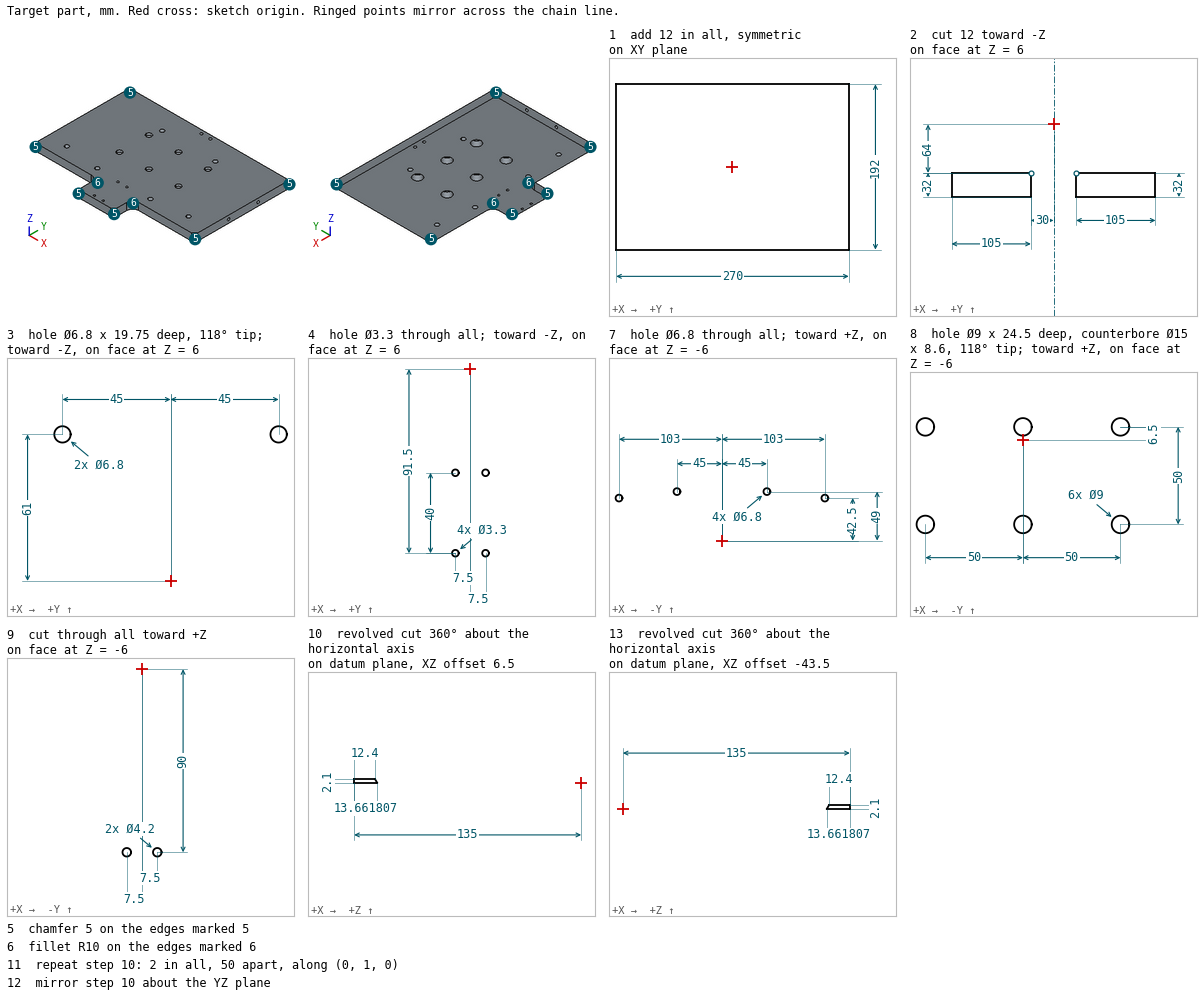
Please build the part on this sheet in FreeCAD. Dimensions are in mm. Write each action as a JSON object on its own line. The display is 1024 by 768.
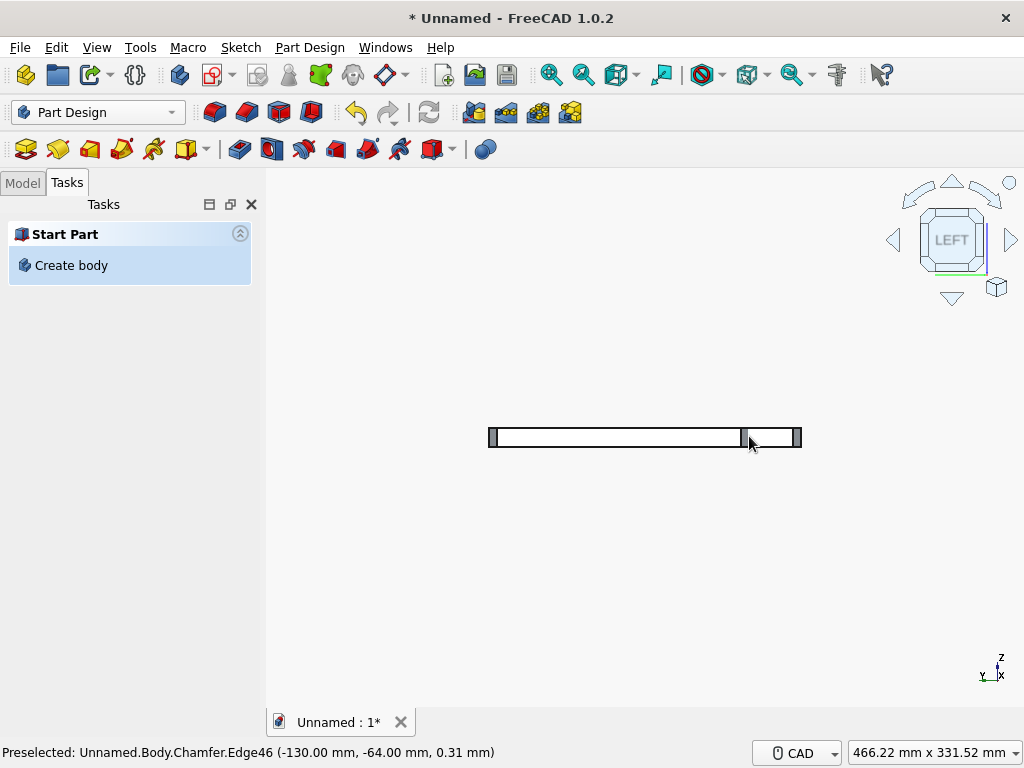
{"action": "key", "text": "v 3"}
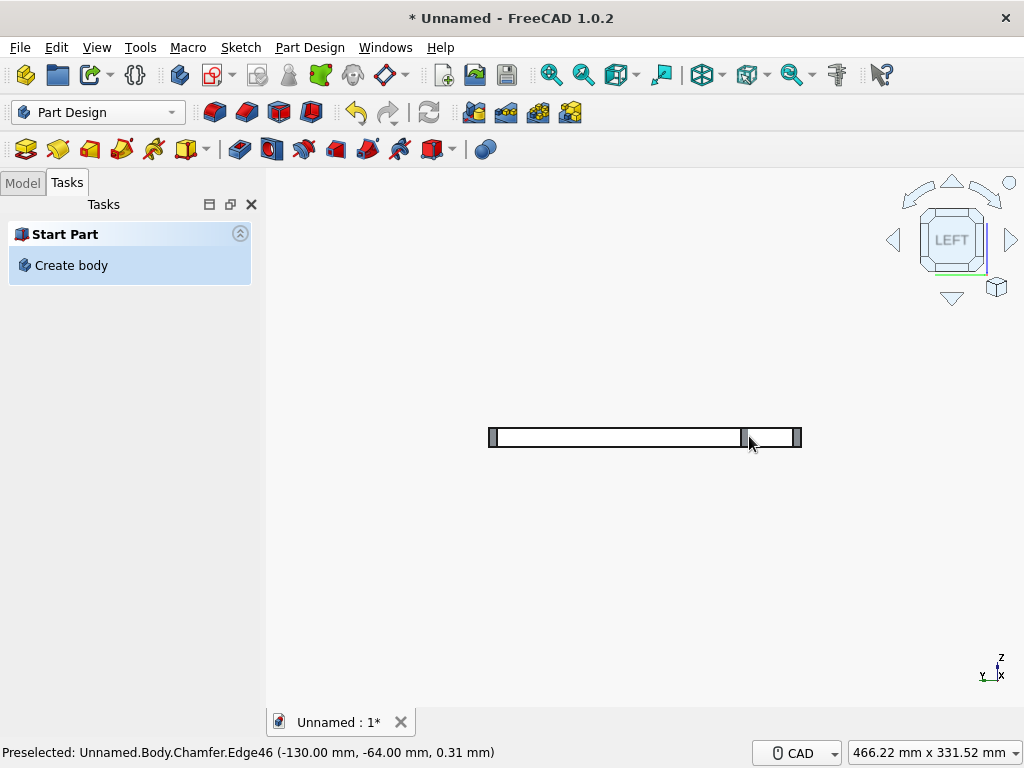
{"action": "key", "text": "0"}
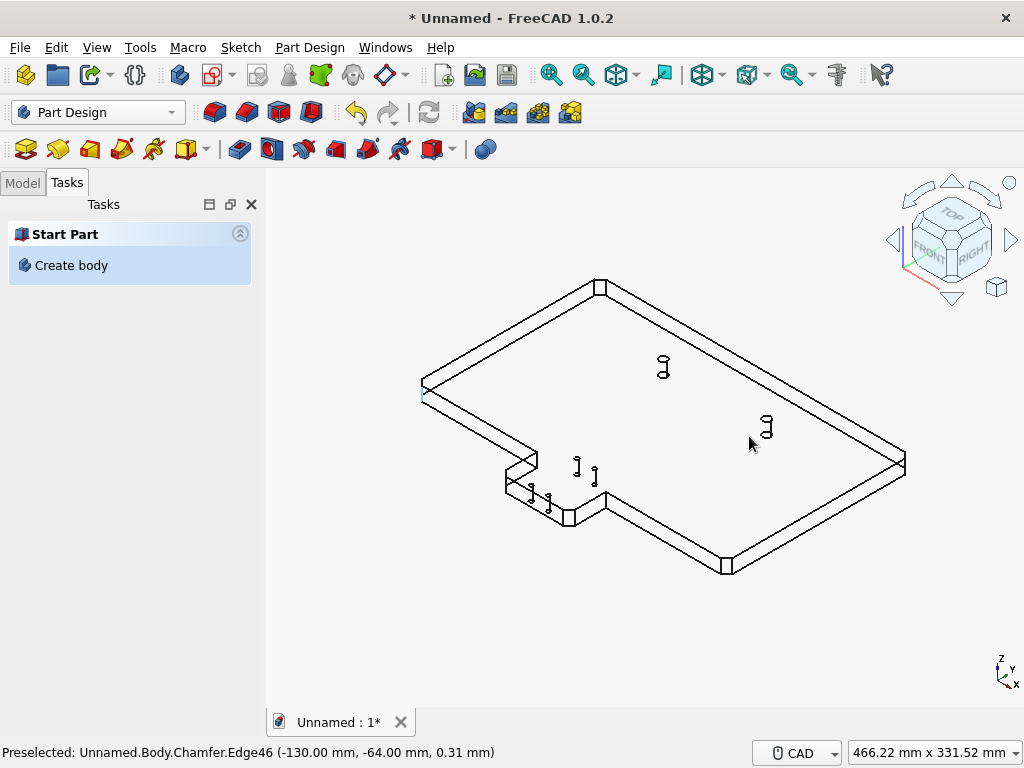
{"action": "left_click", "coordinate": [537, 459]}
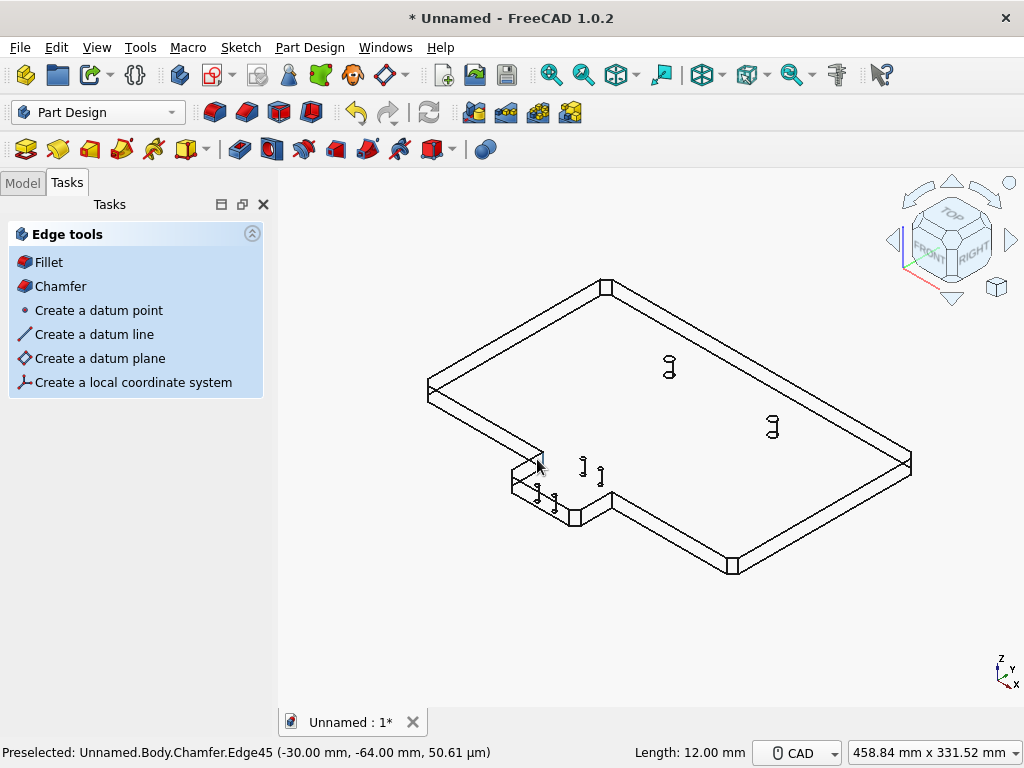
{"action": "left_click", "coordinate": [612, 499], "text": "ctrl"}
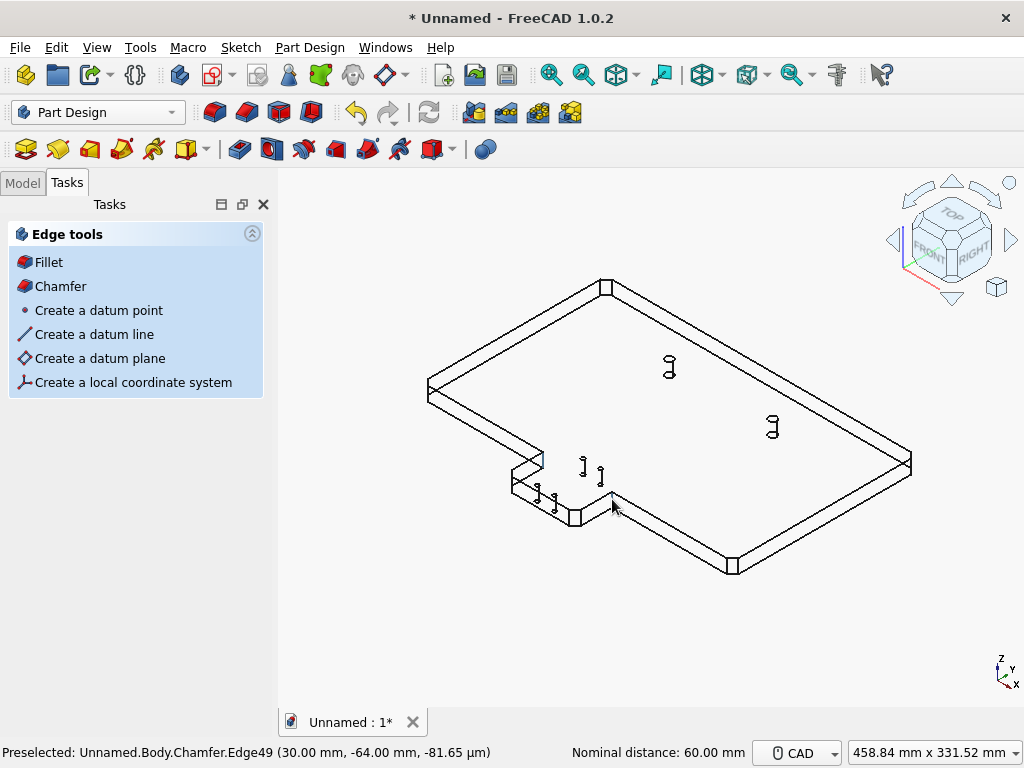
{"action": "key", "text": "v 1"}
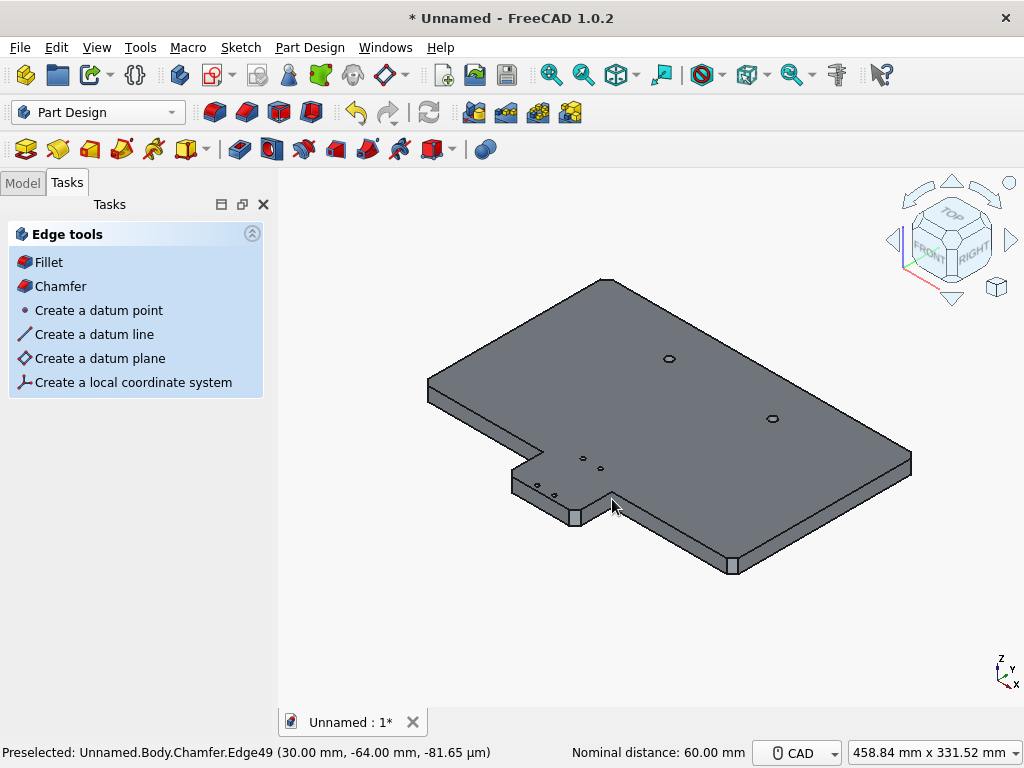
{"action": "left_click", "coordinate": [216, 112]}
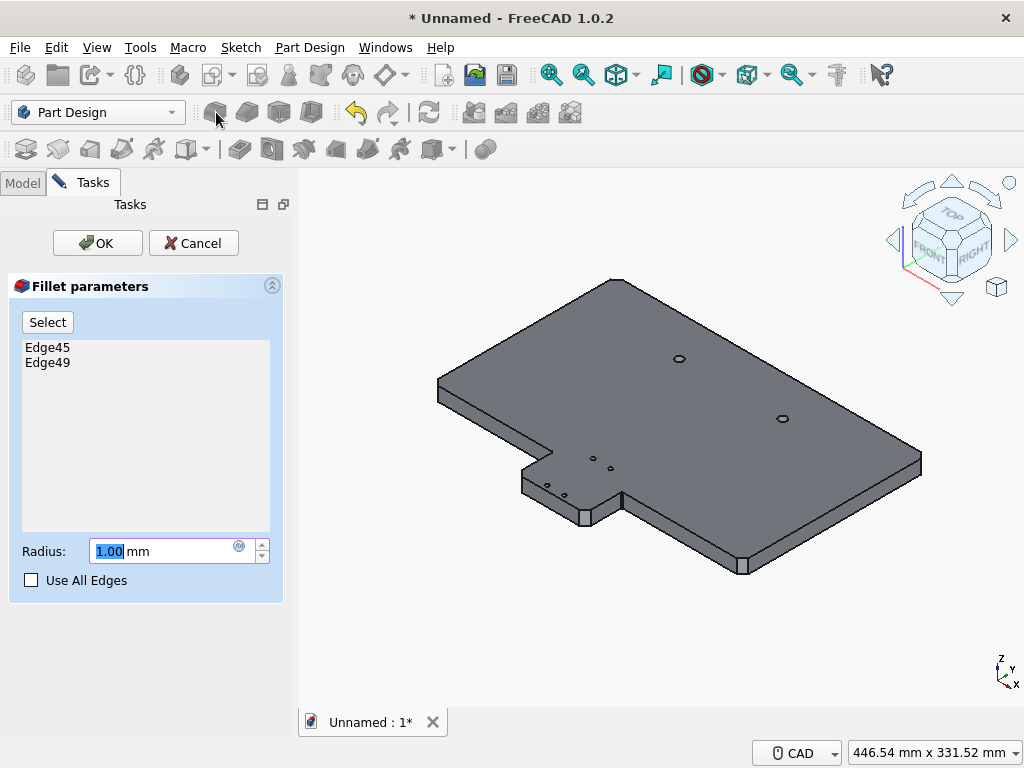
{"action": "type", "text": "10"}
{"action": "key", "text": "Tab"}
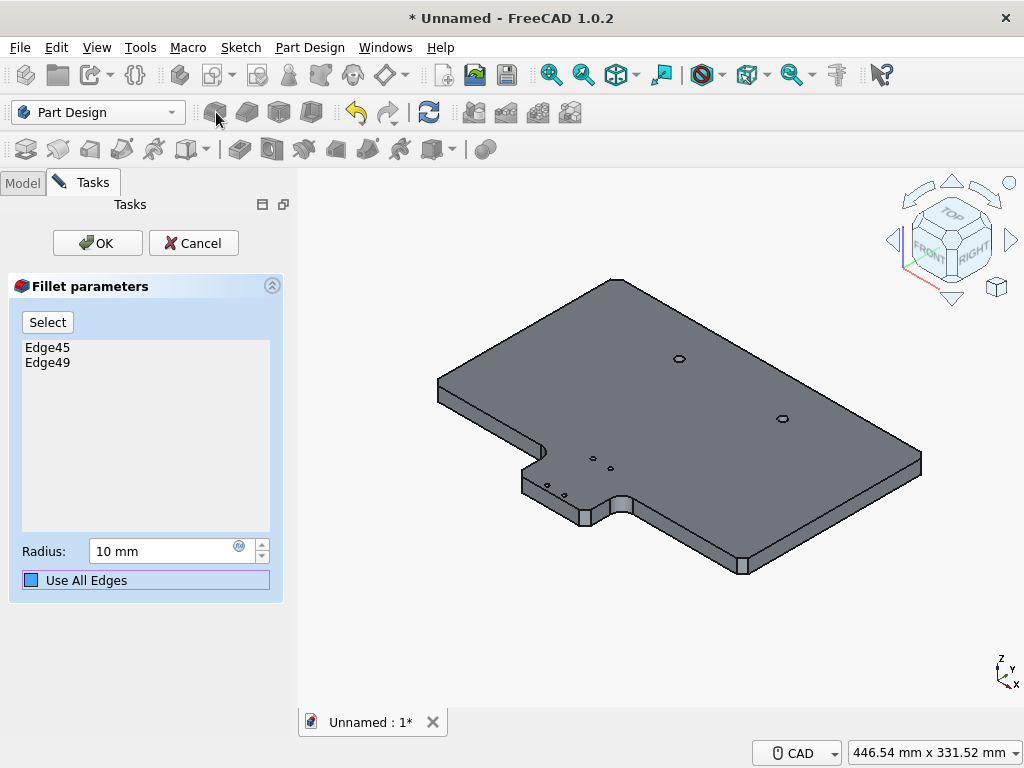
{"action": "left_click", "coordinate": [98, 243]}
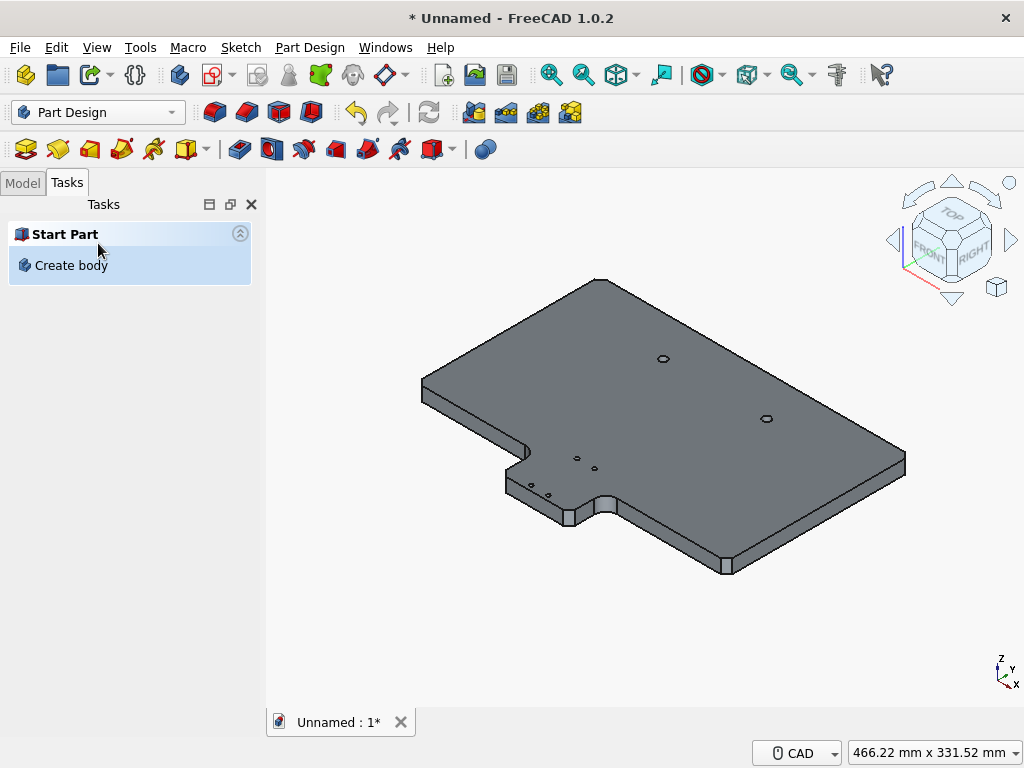
{"action": "key", "text": "5"}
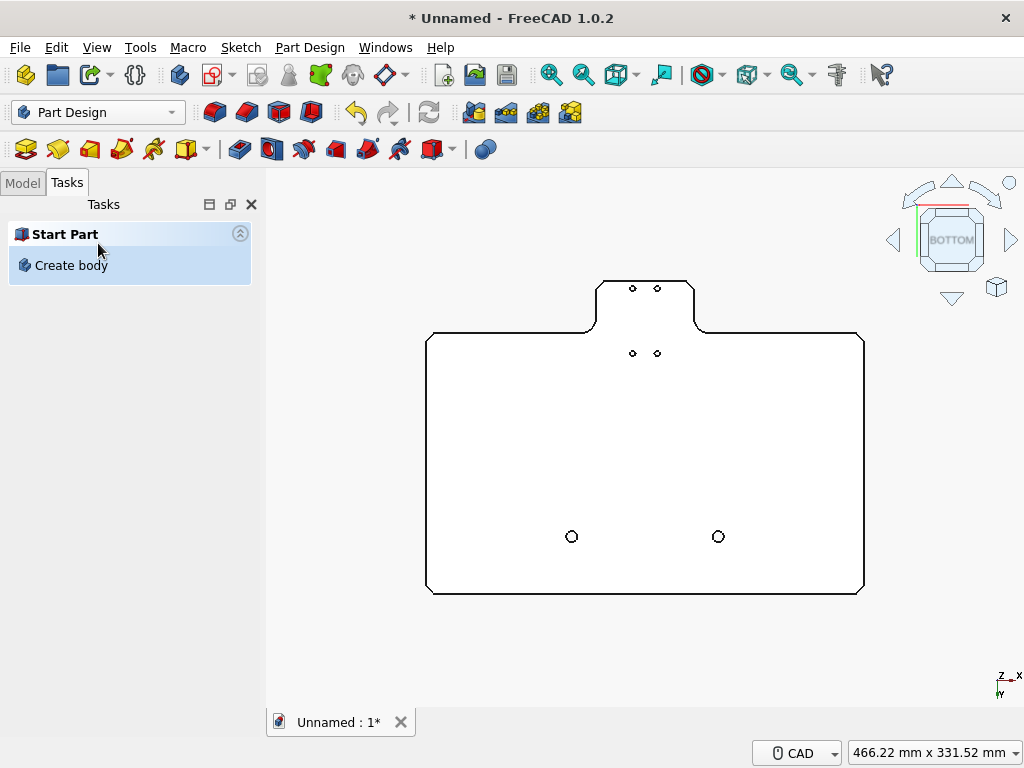
{"action": "left_click", "coordinate": [582, 436]}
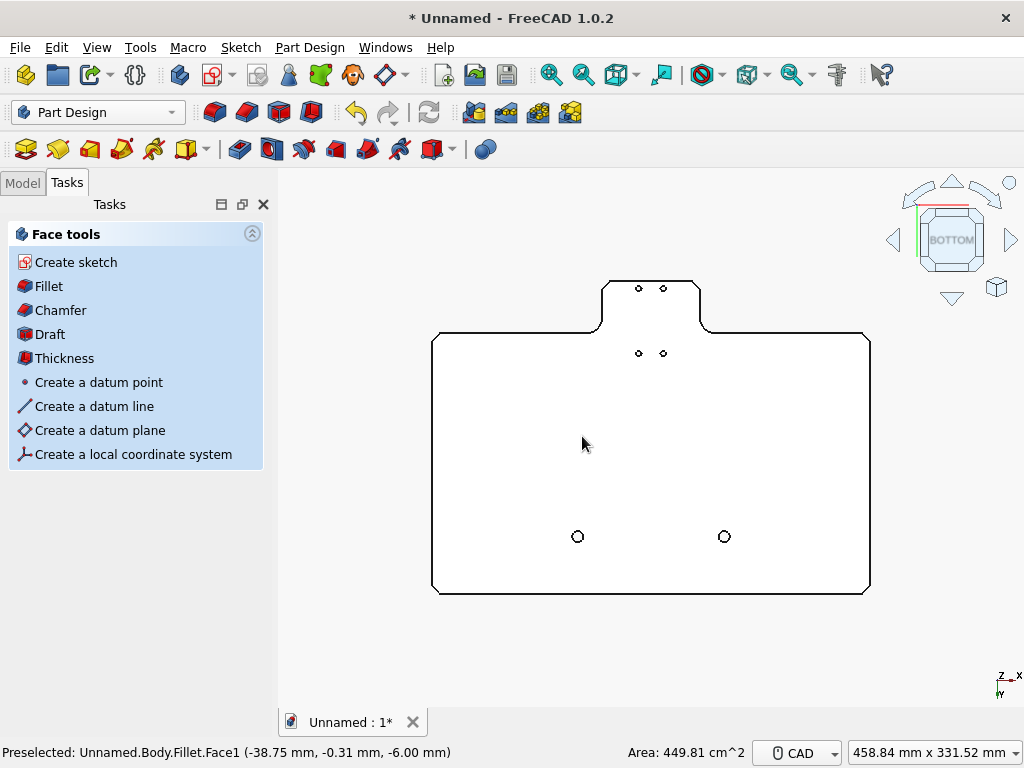
{"action": "left_click", "coordinate": [212, 76]}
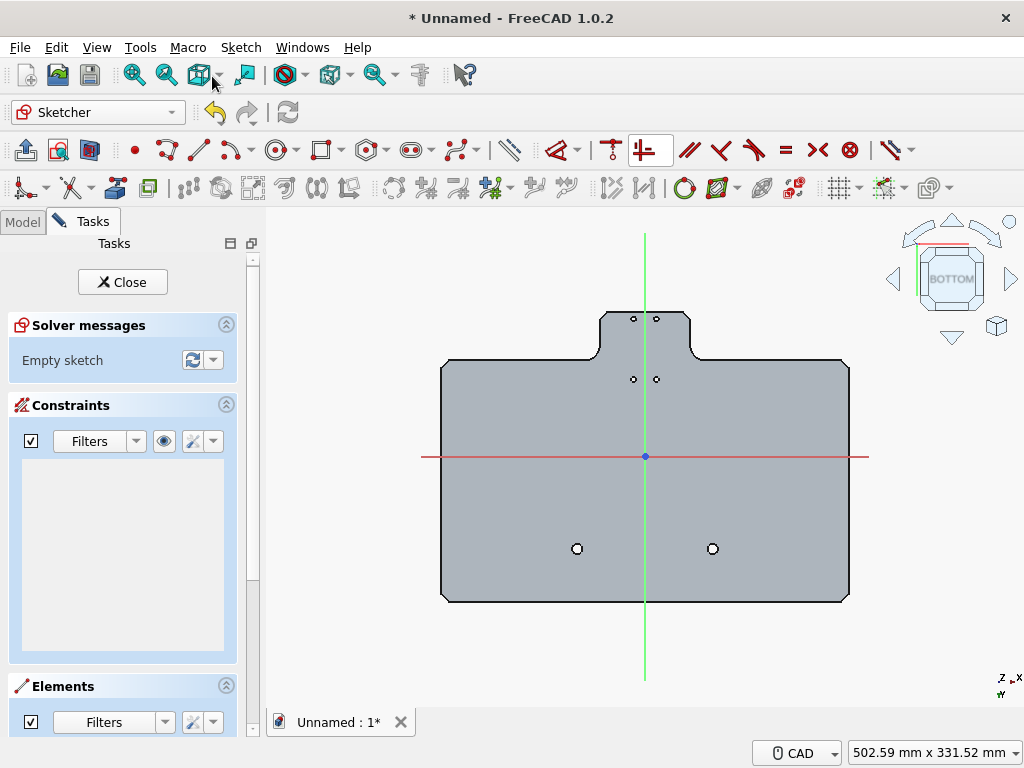
{"action": "key", "text": "g c"}